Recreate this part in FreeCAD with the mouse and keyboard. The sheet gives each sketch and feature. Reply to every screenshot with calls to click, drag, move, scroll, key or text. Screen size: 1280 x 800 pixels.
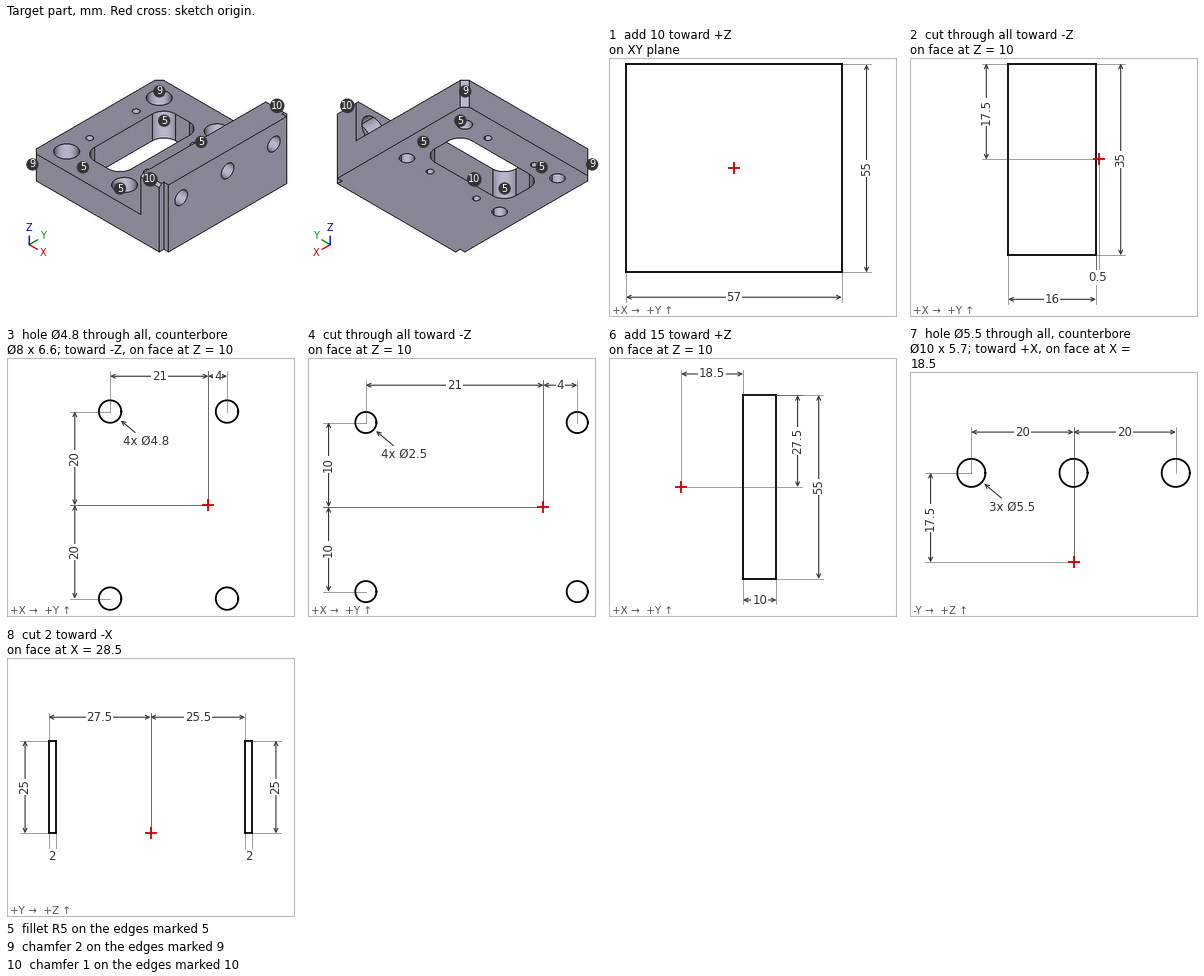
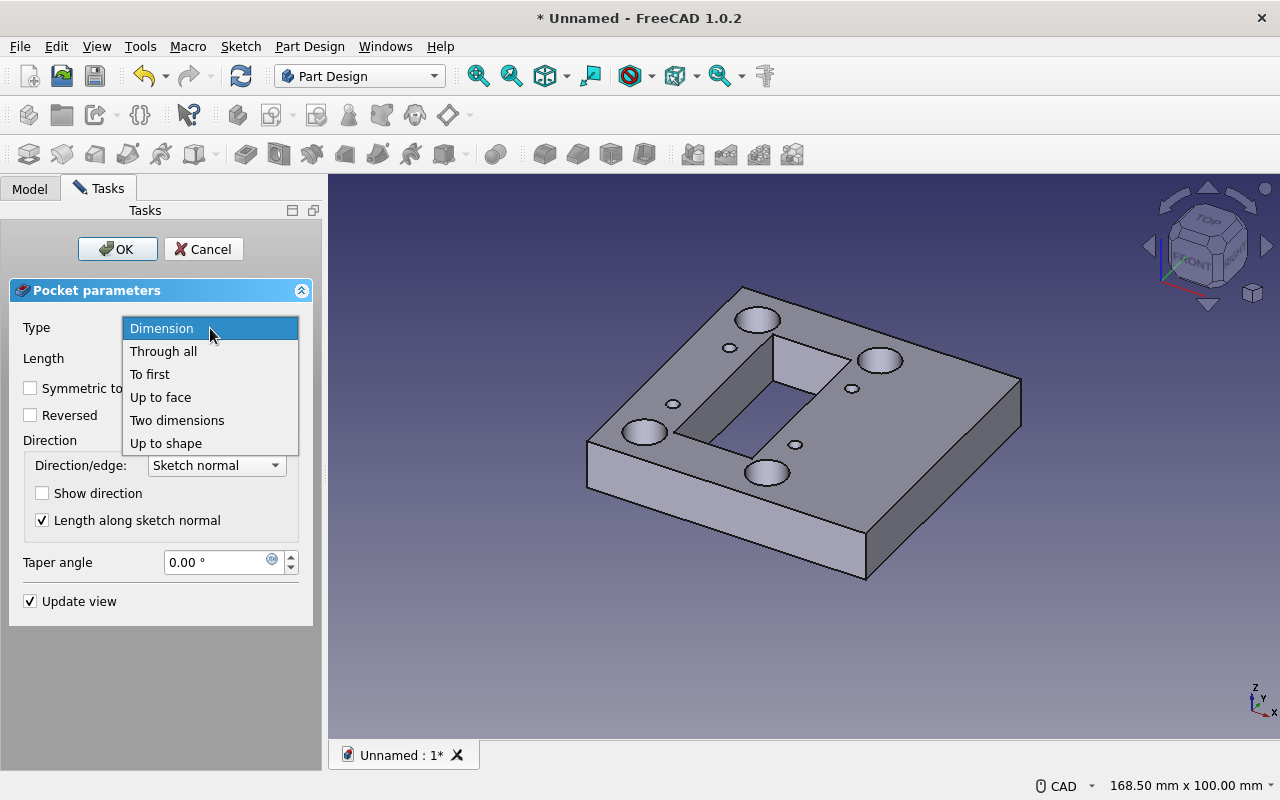
click(208, 352)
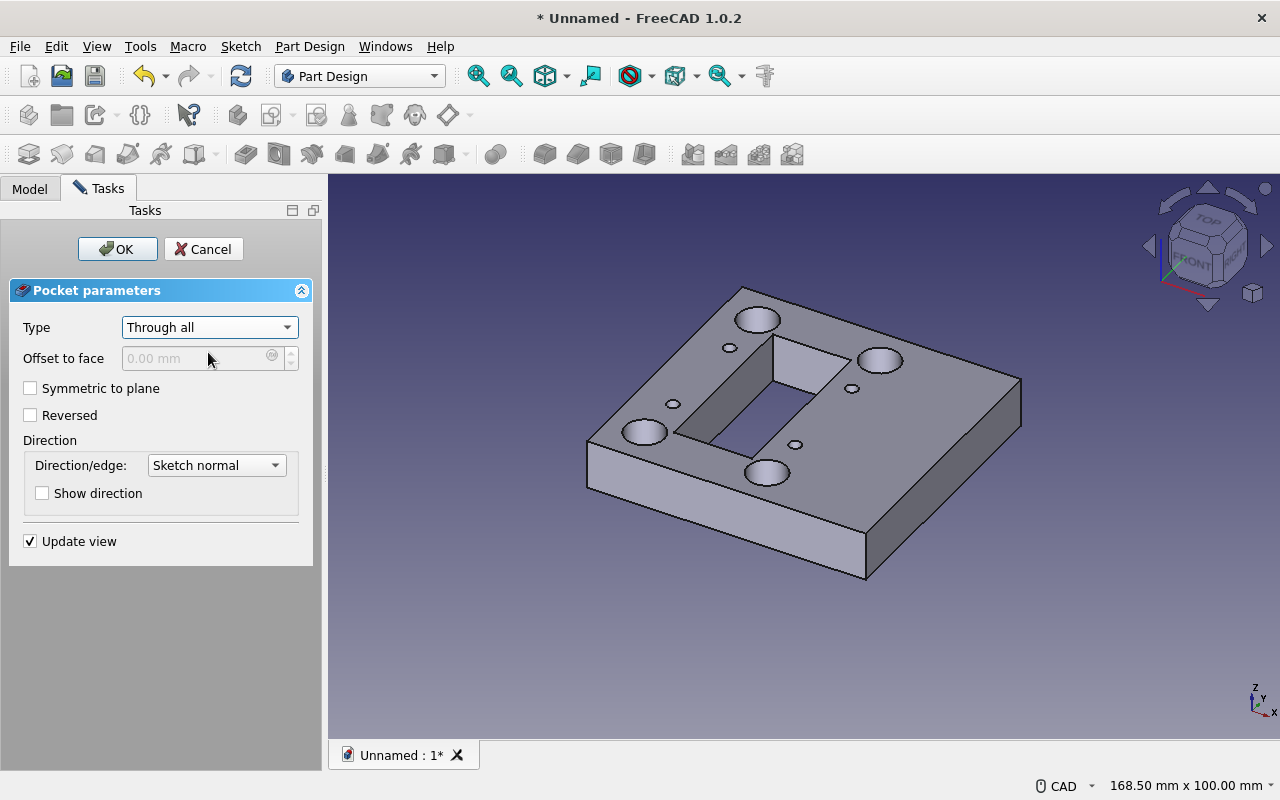
click(118, 249)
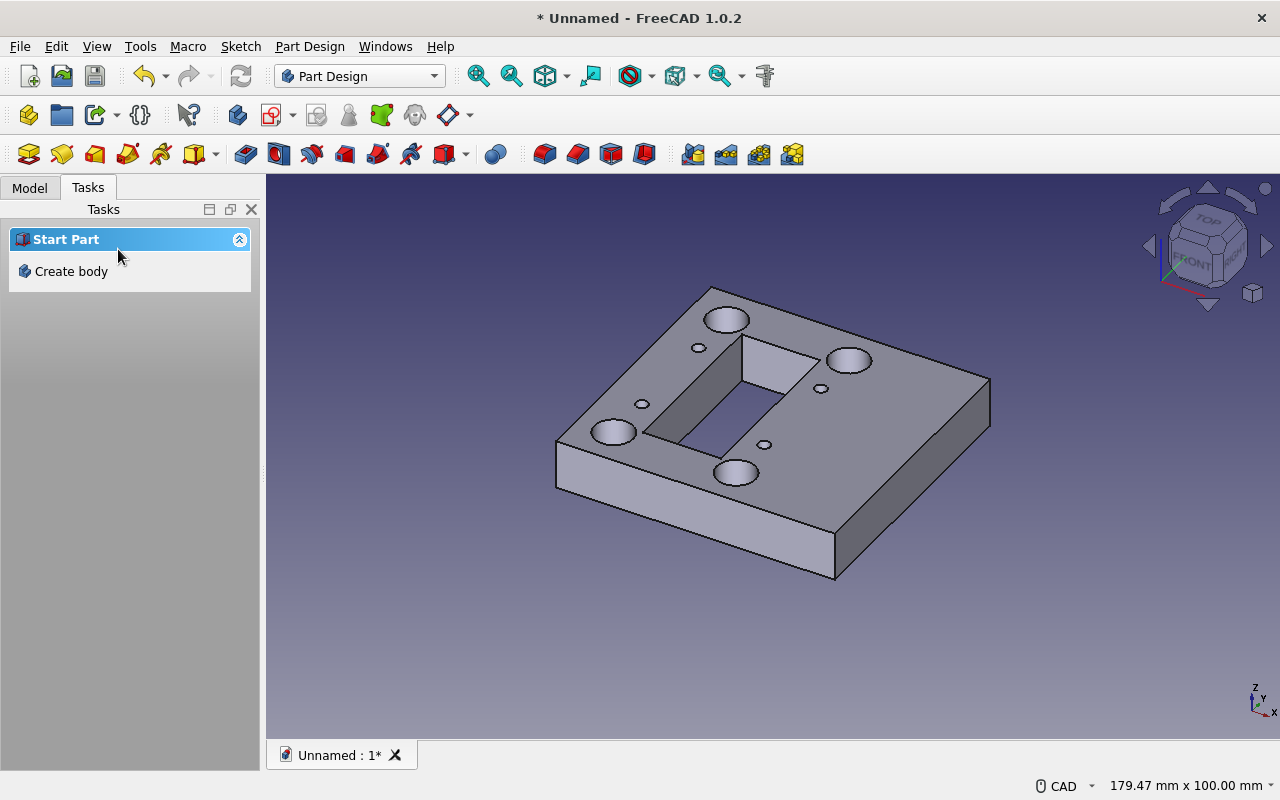
key(0)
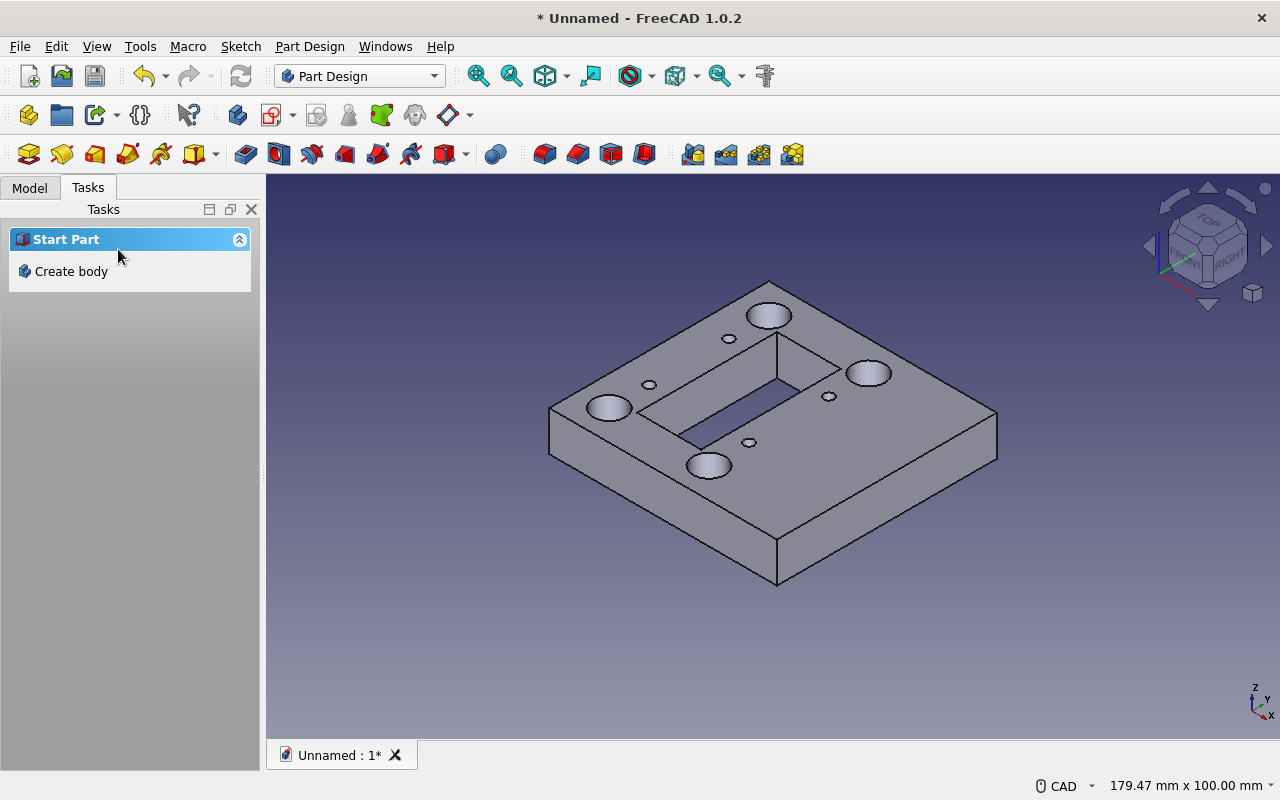
key(2)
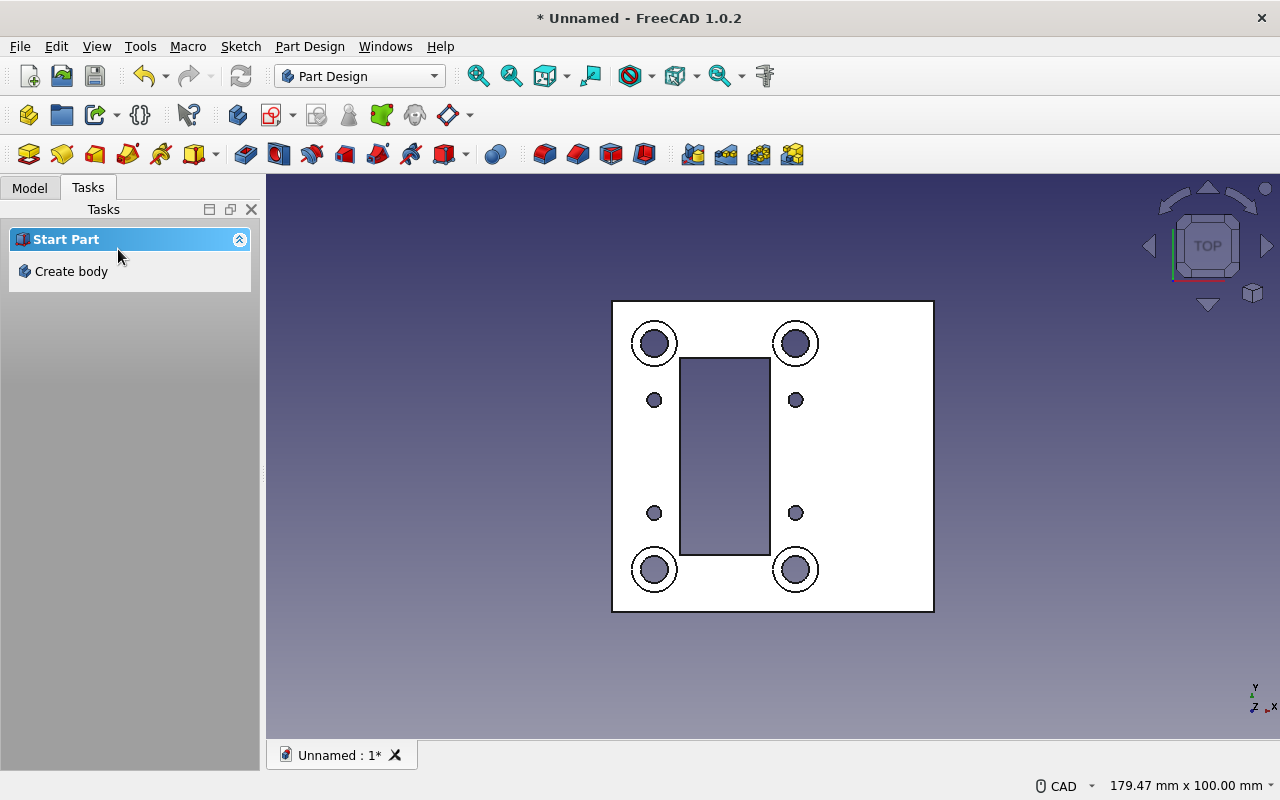
key(1)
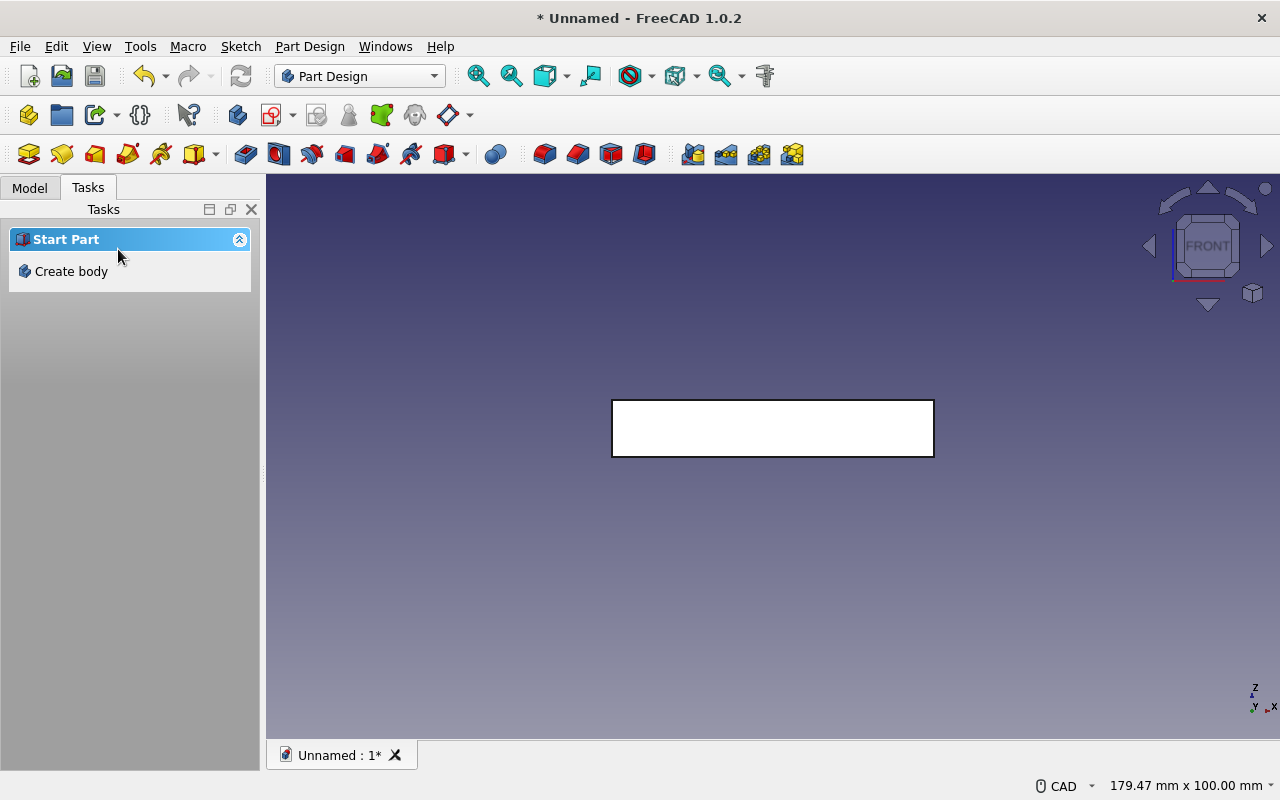
click(479, 76)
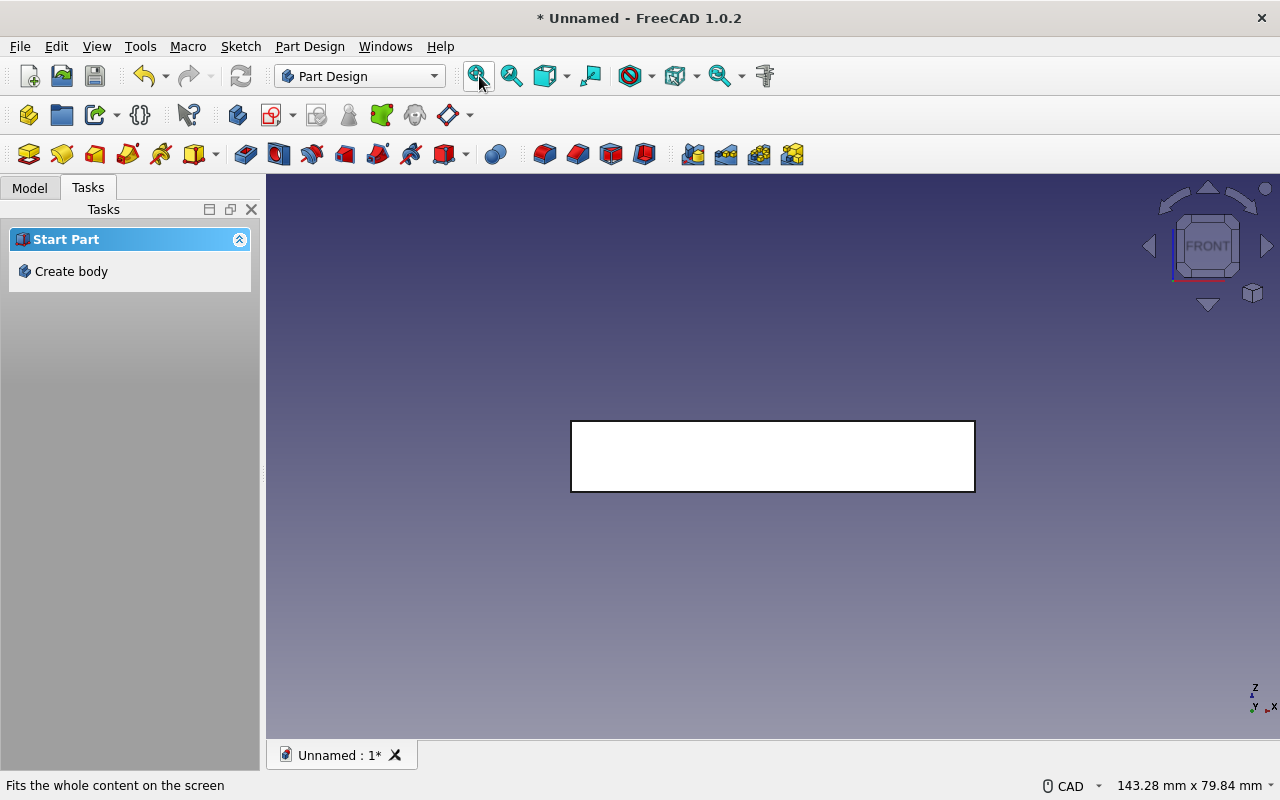
key(3)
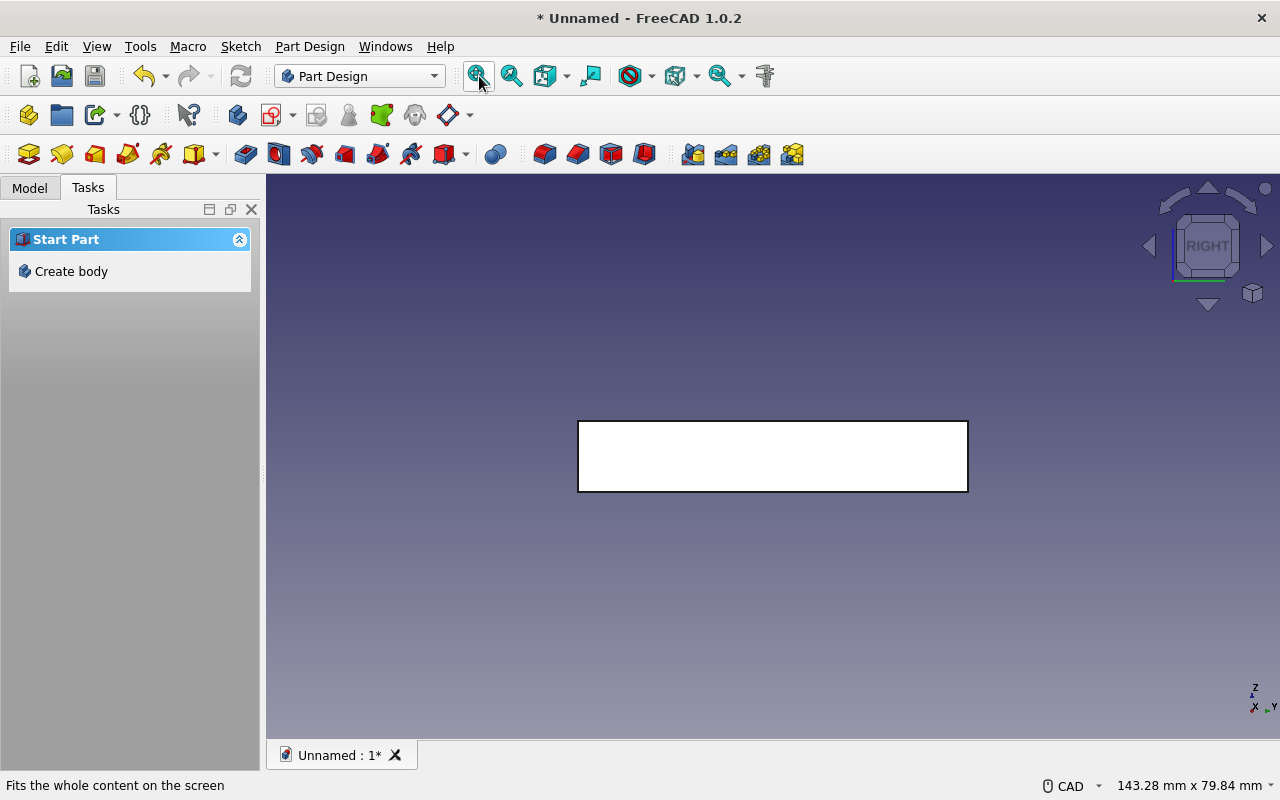
click(479, 76)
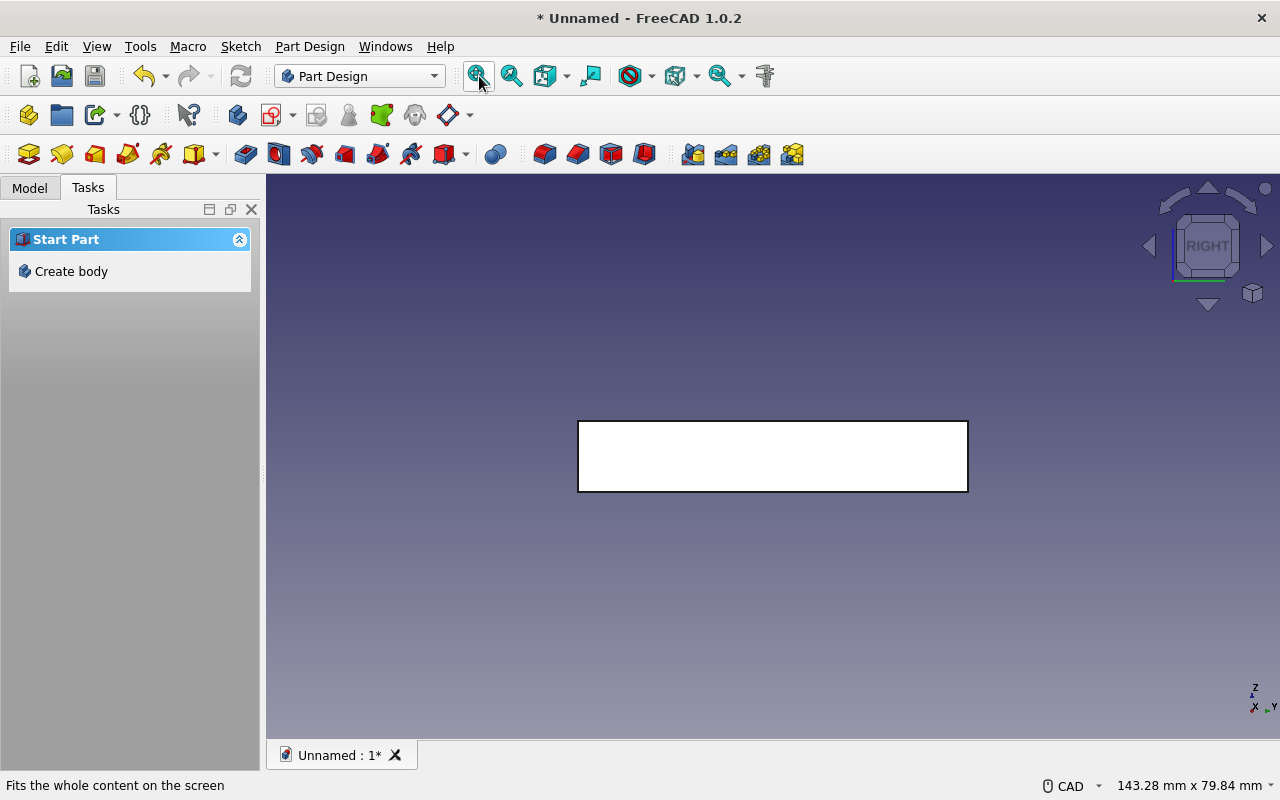
key(5)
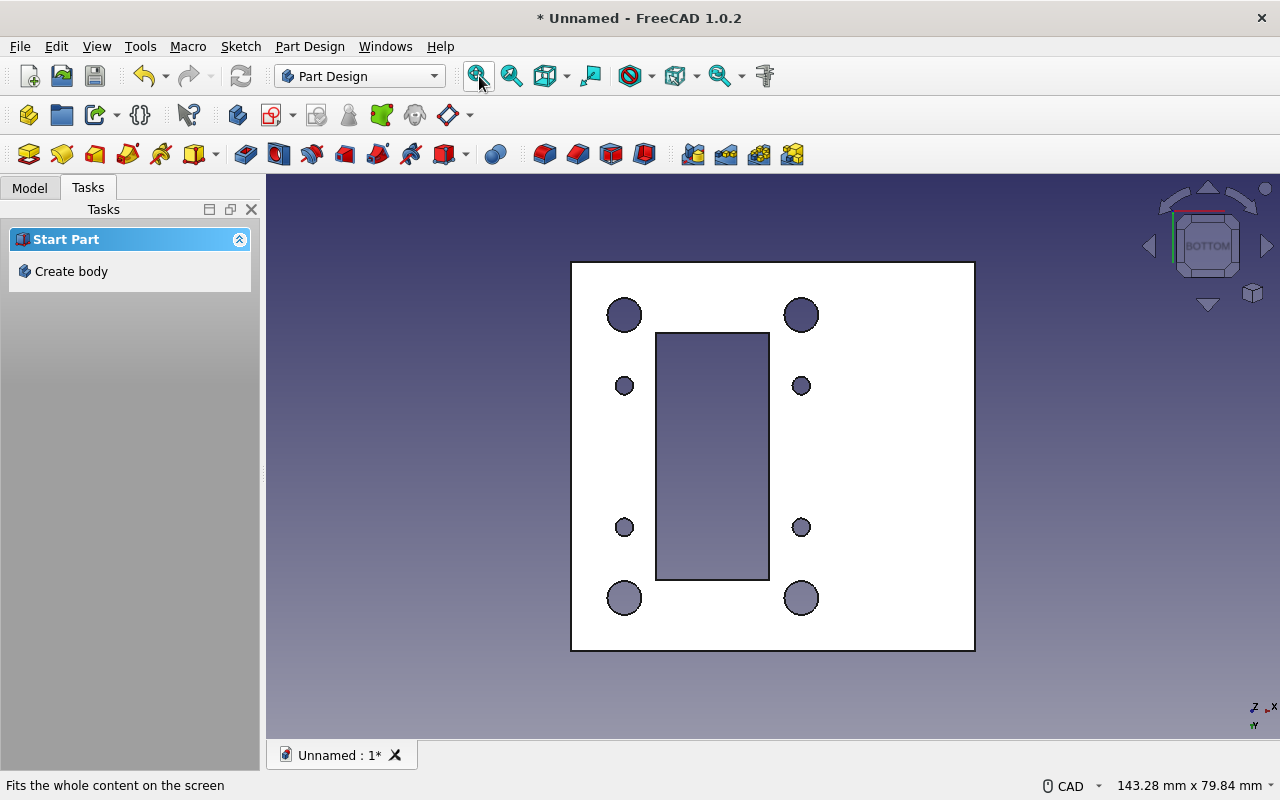
key(4)